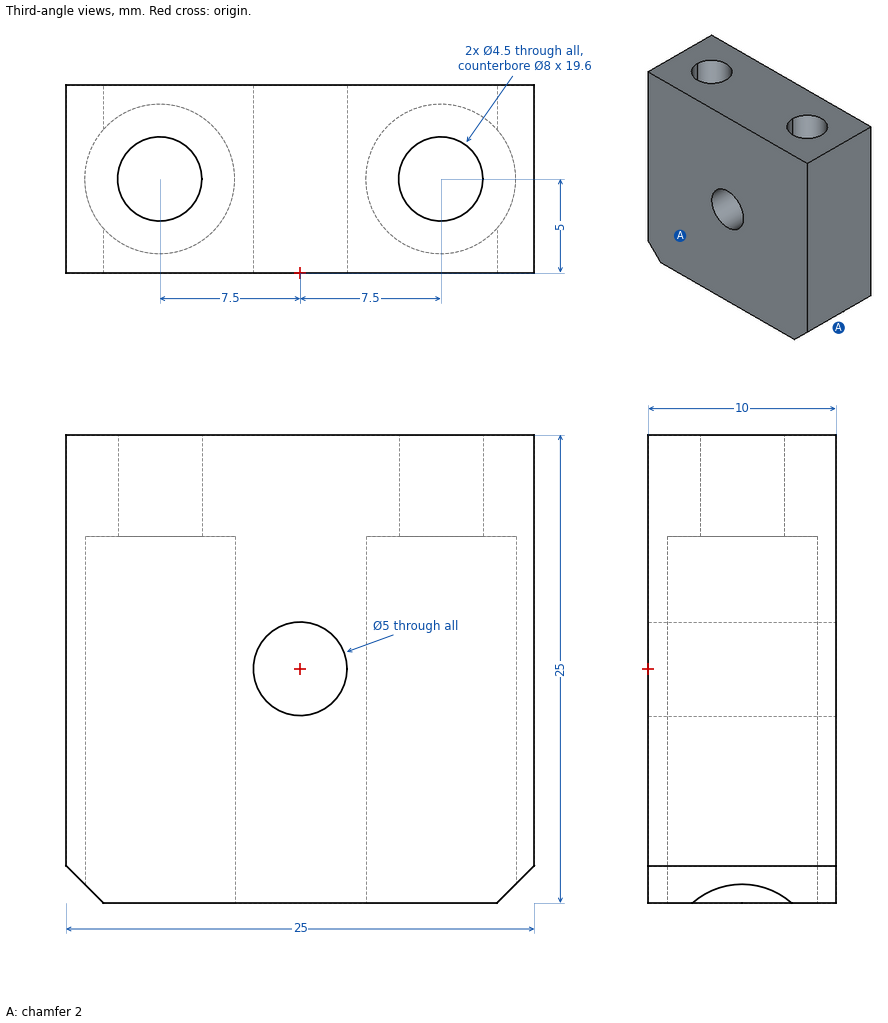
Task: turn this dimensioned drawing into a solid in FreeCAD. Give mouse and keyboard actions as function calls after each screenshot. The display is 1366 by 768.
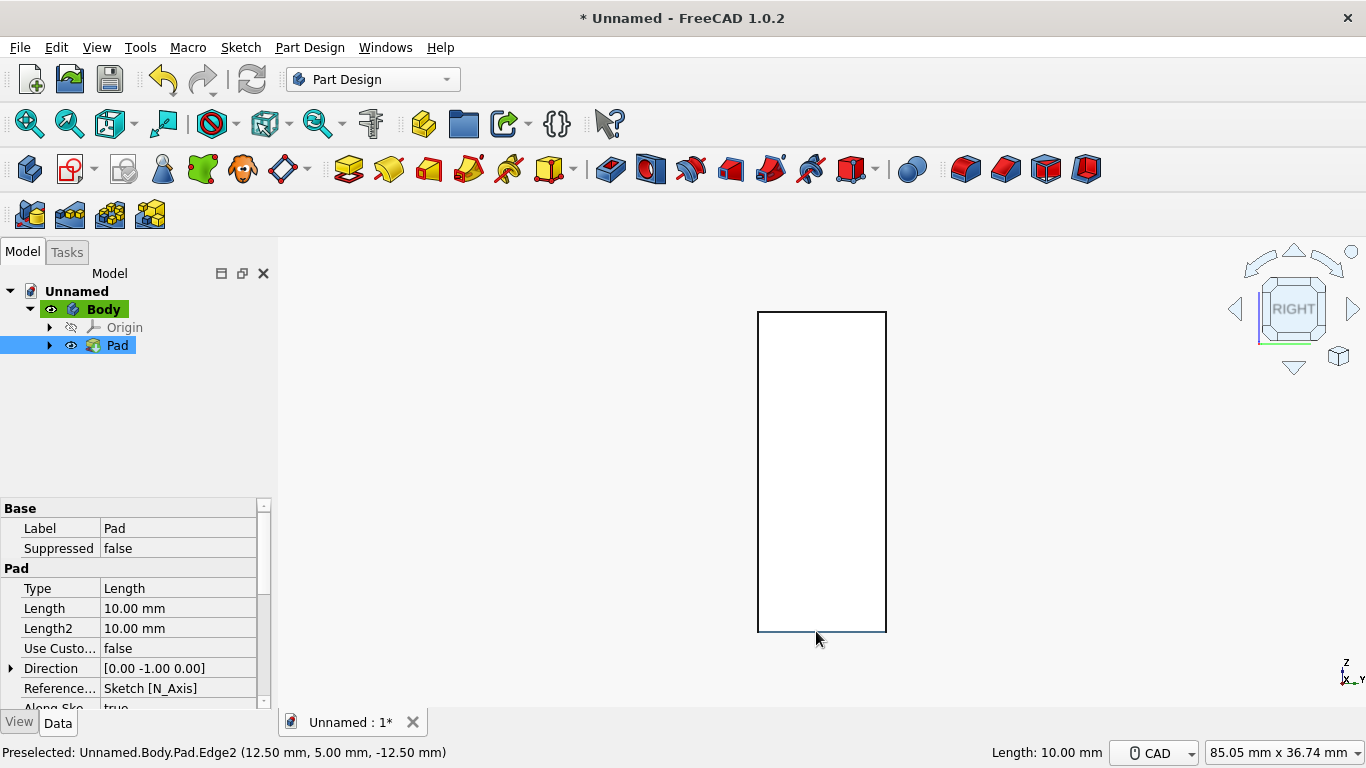
key(5)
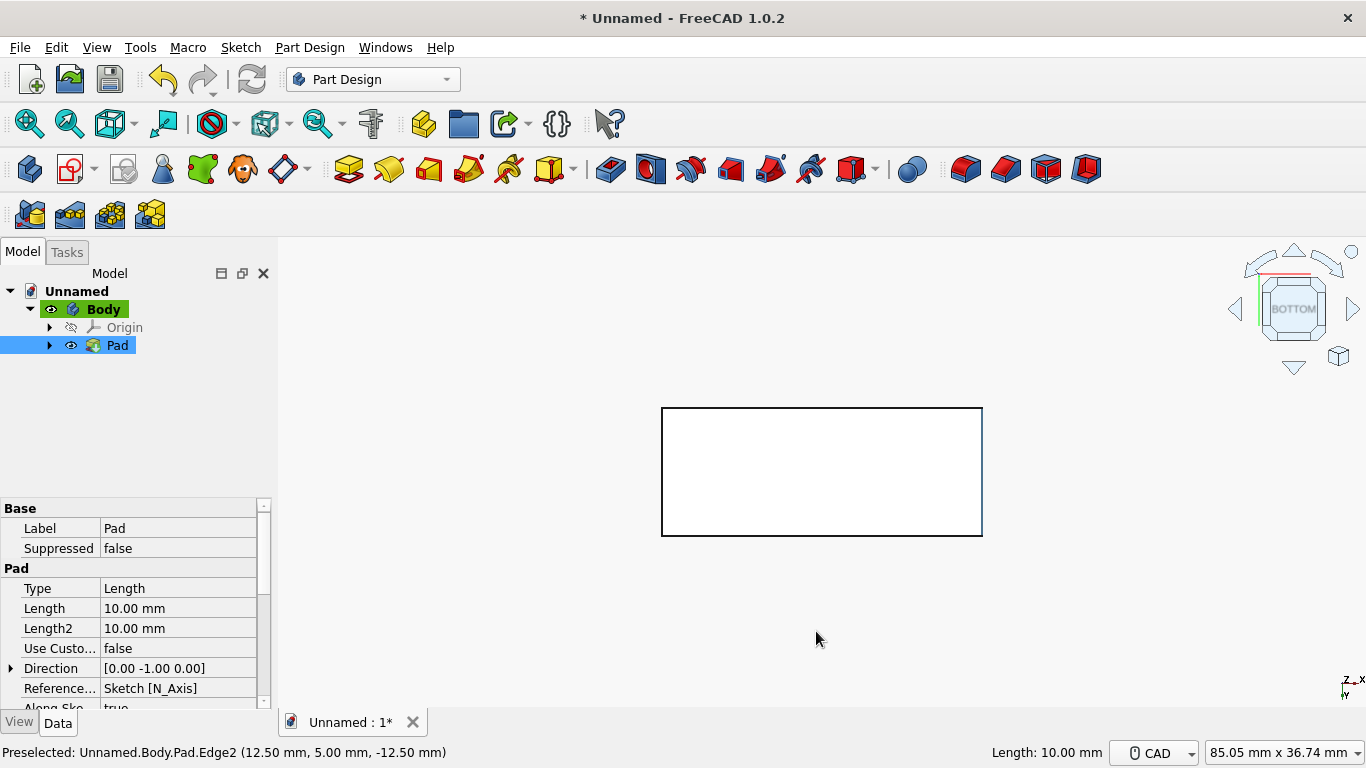
key(v)
key(f)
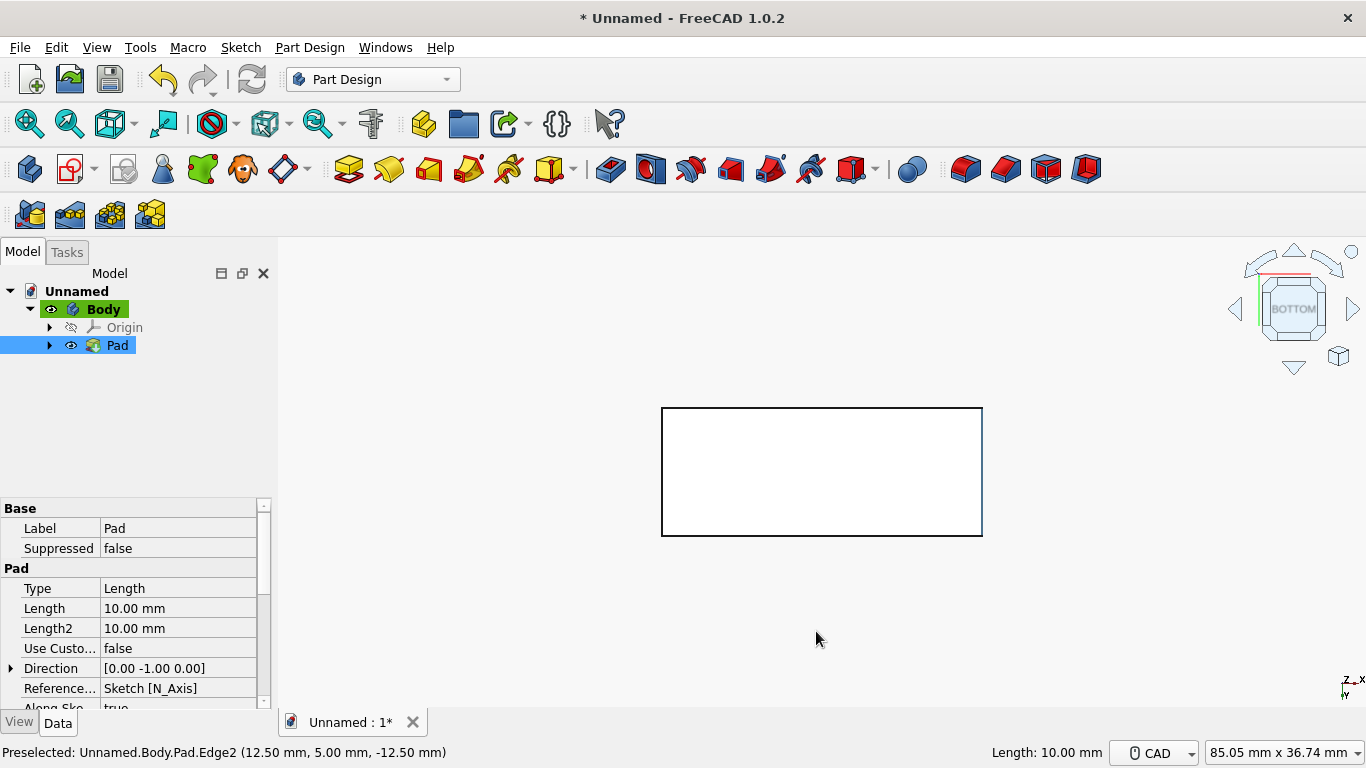
click(662, 471, ctrl)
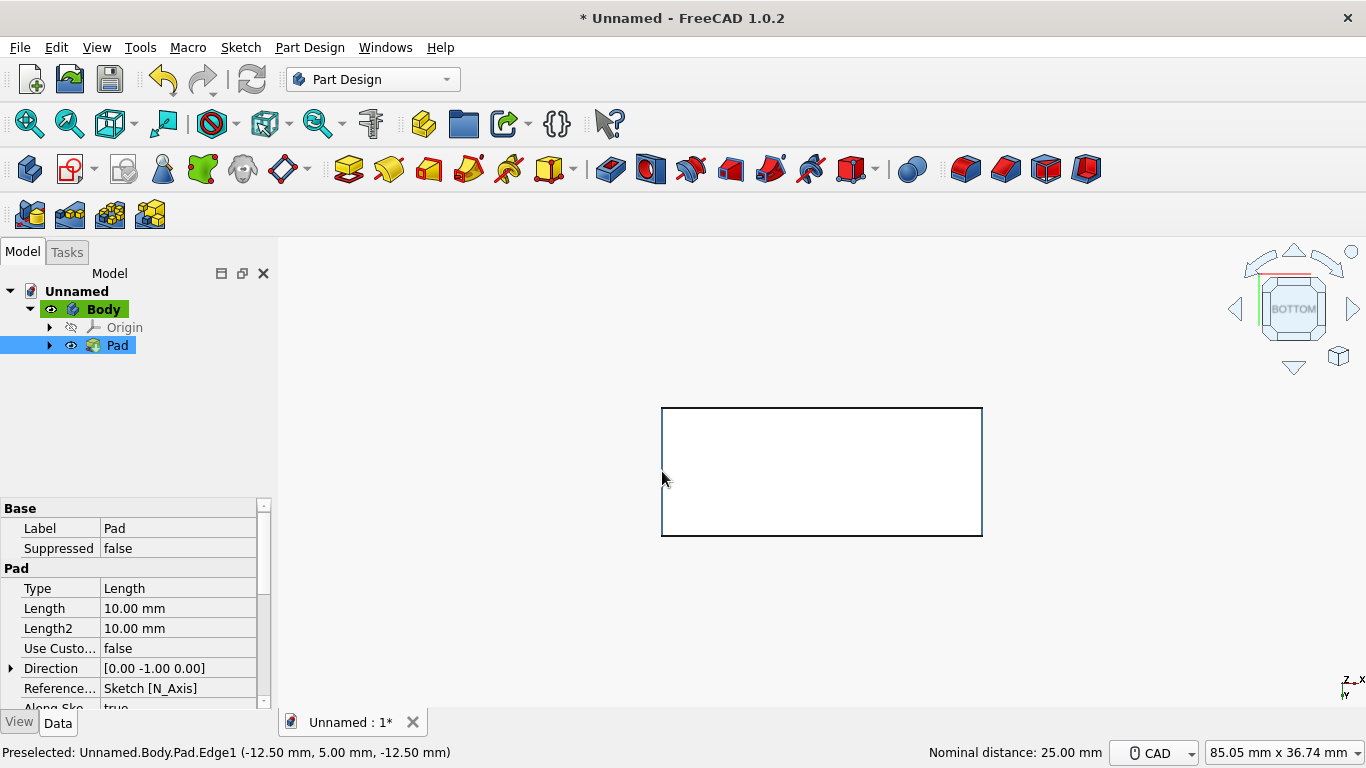
click(1006, 170)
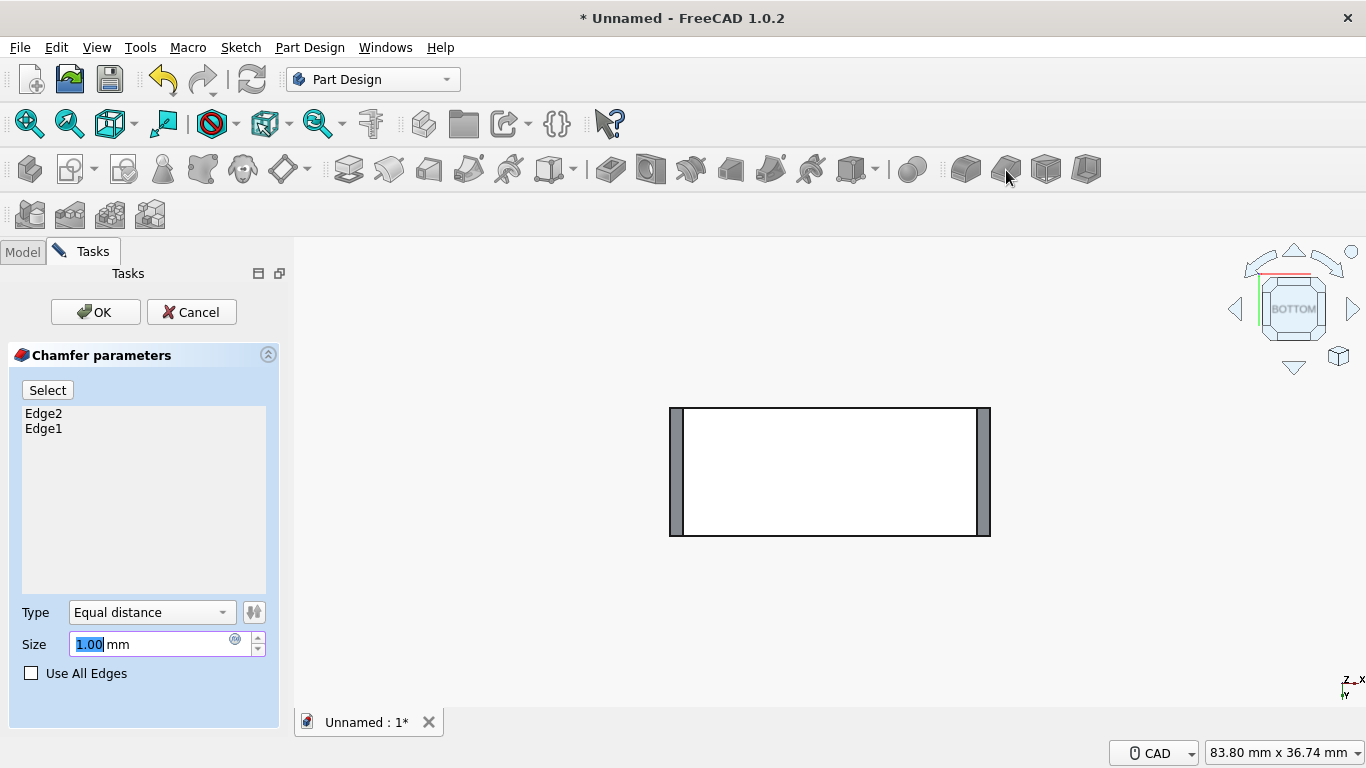
text(2)
key(Tab)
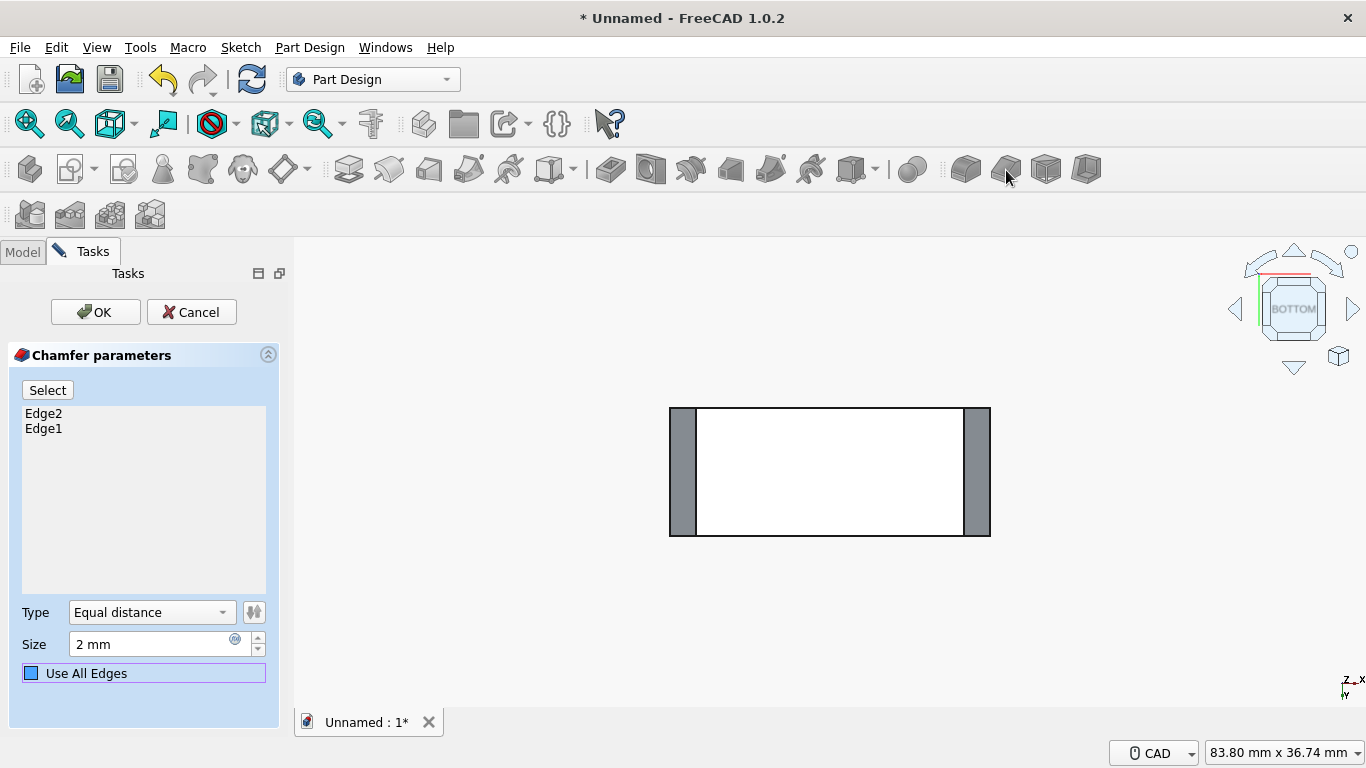
click(96, 312)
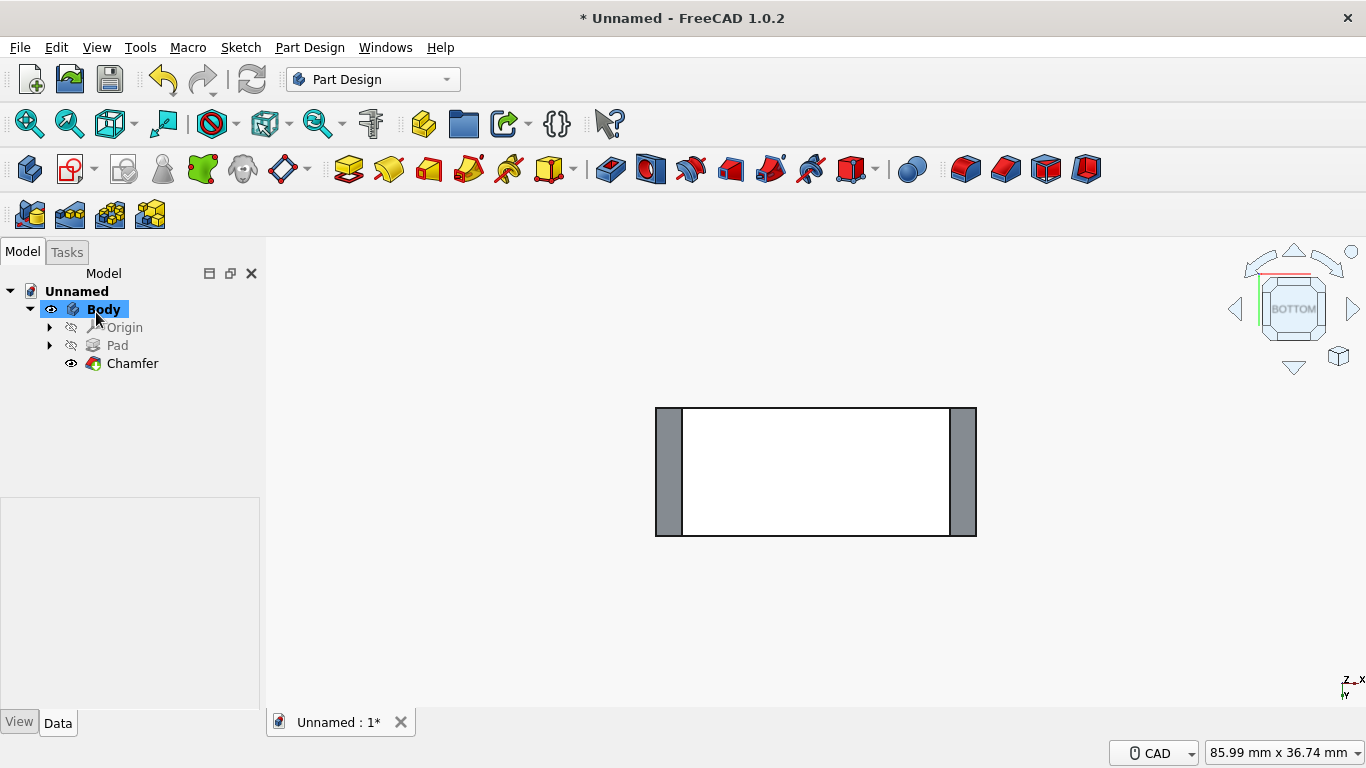
key(v)
key(f)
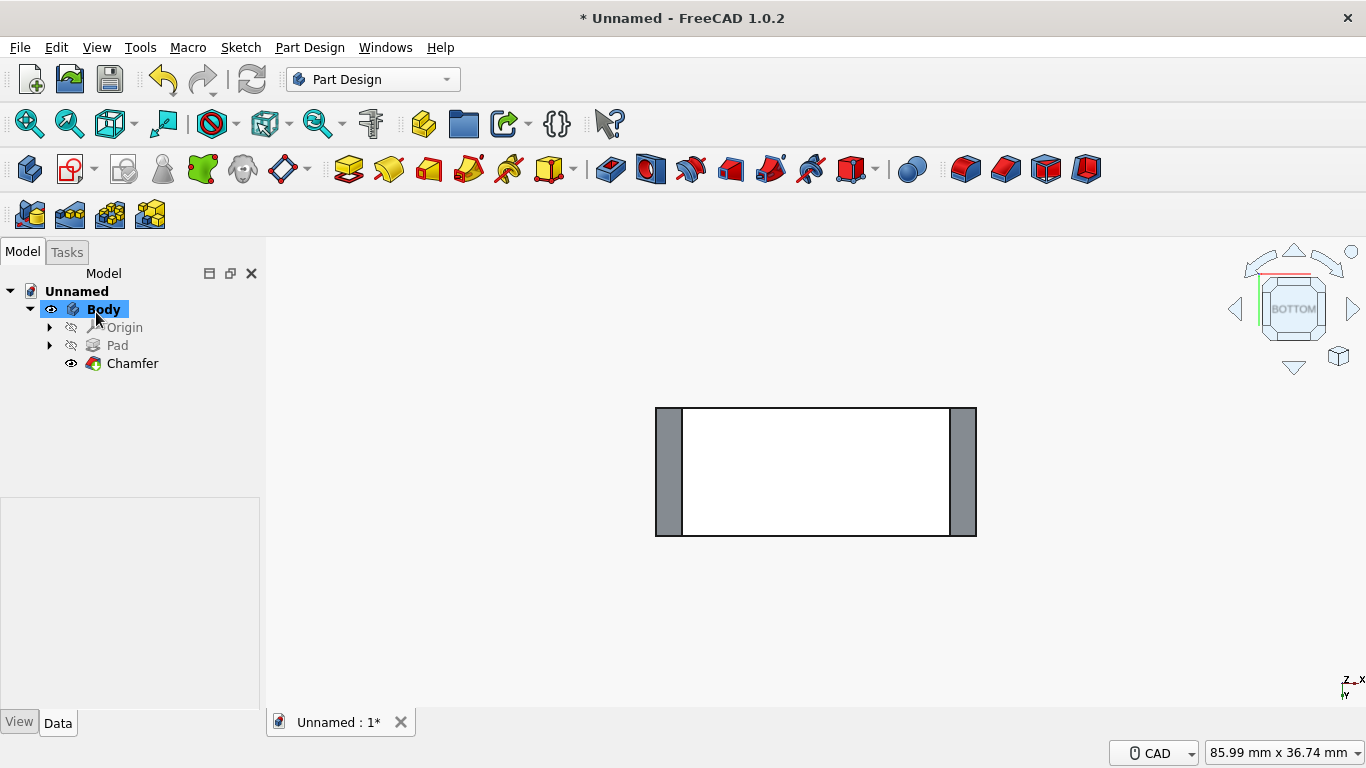
click(70, 170)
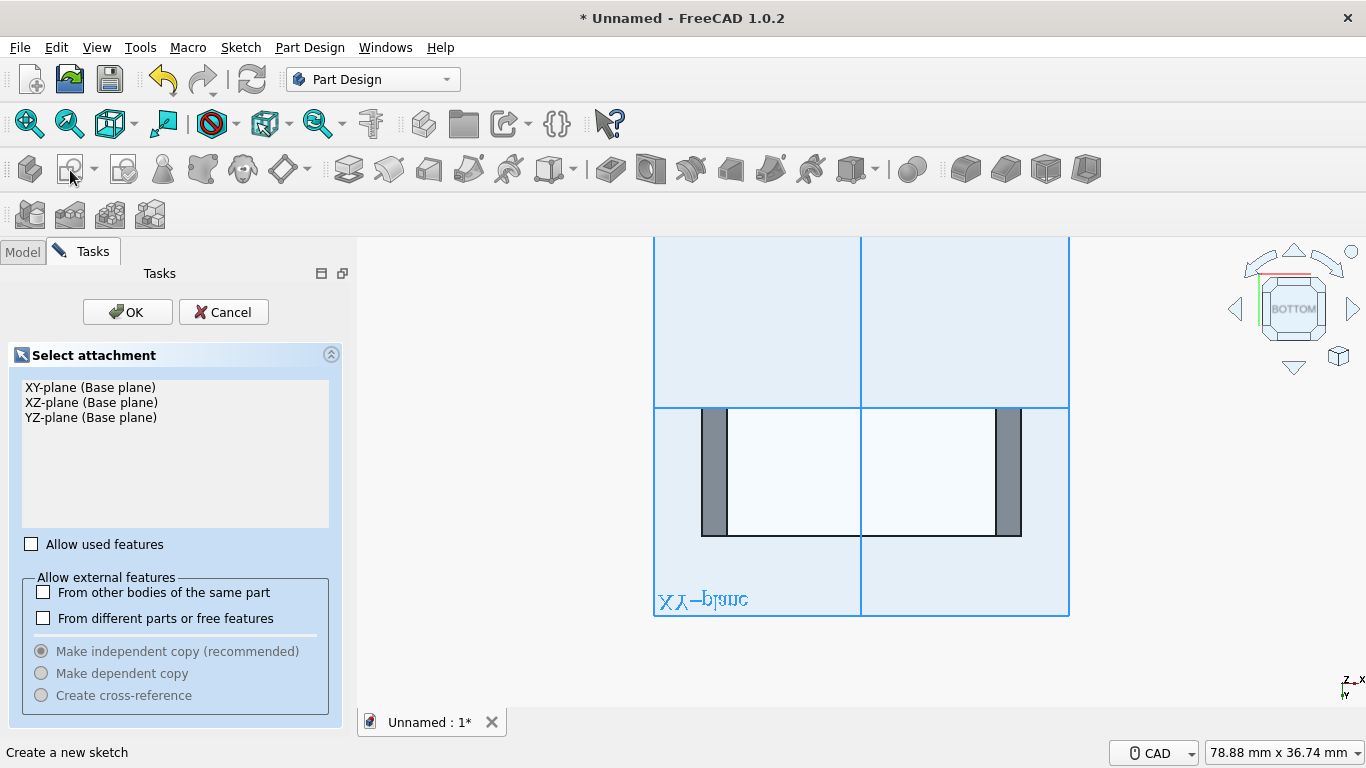
click(82, 402)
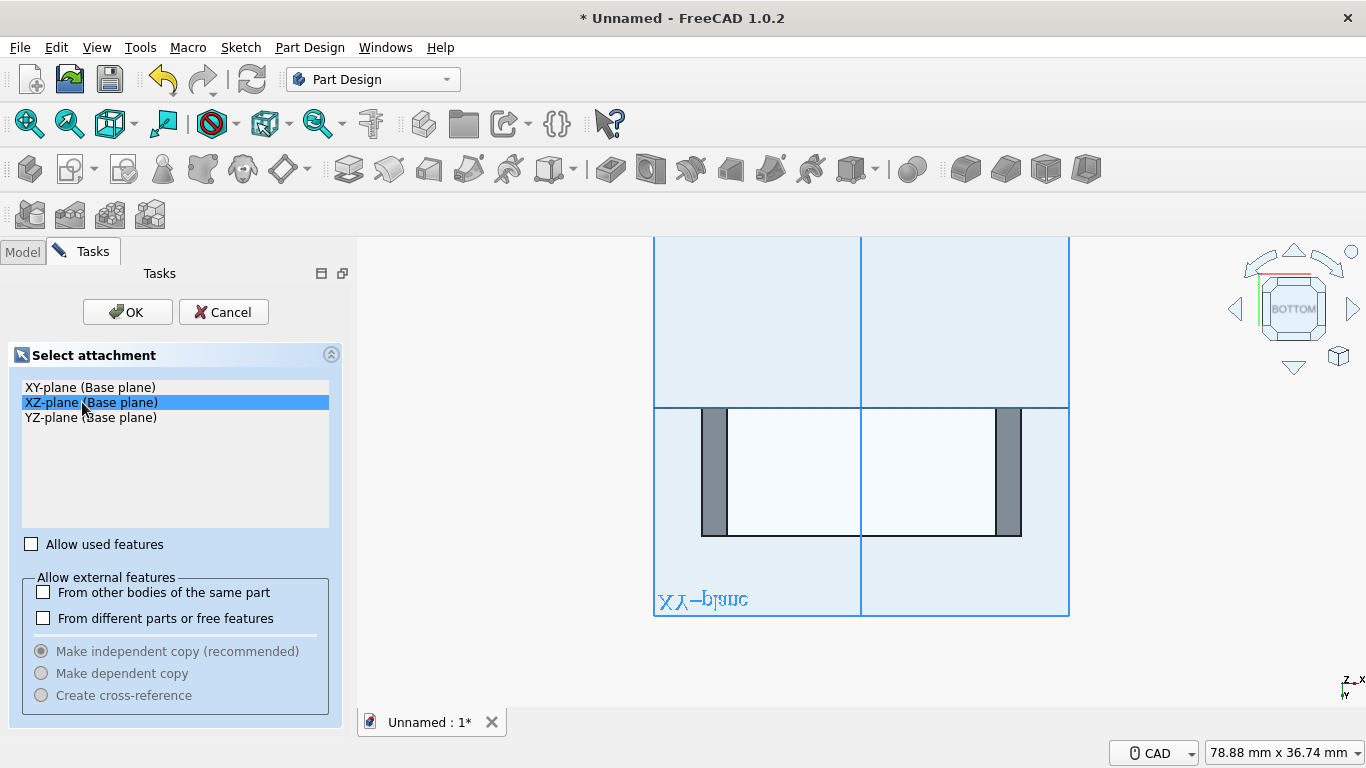
click(128, 312)